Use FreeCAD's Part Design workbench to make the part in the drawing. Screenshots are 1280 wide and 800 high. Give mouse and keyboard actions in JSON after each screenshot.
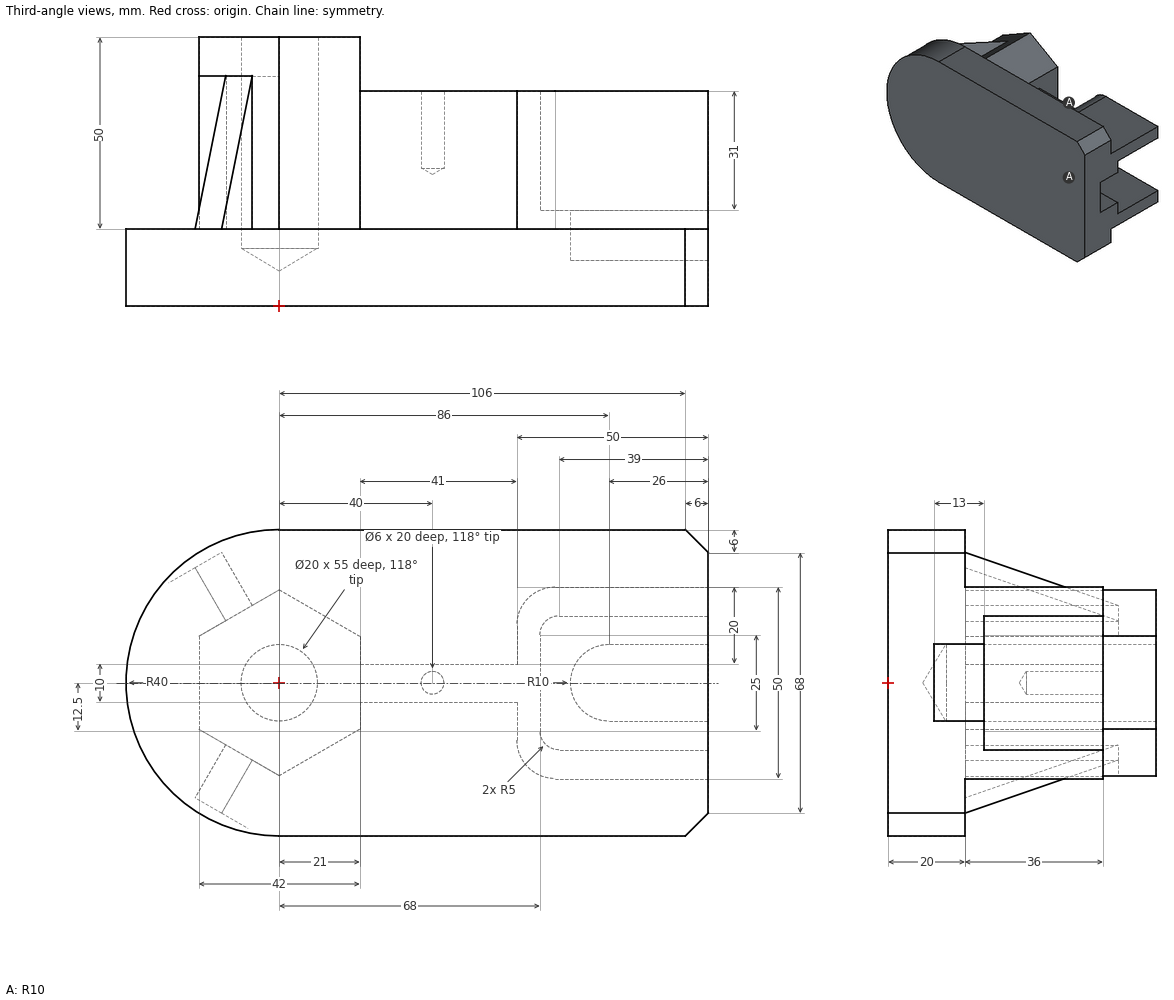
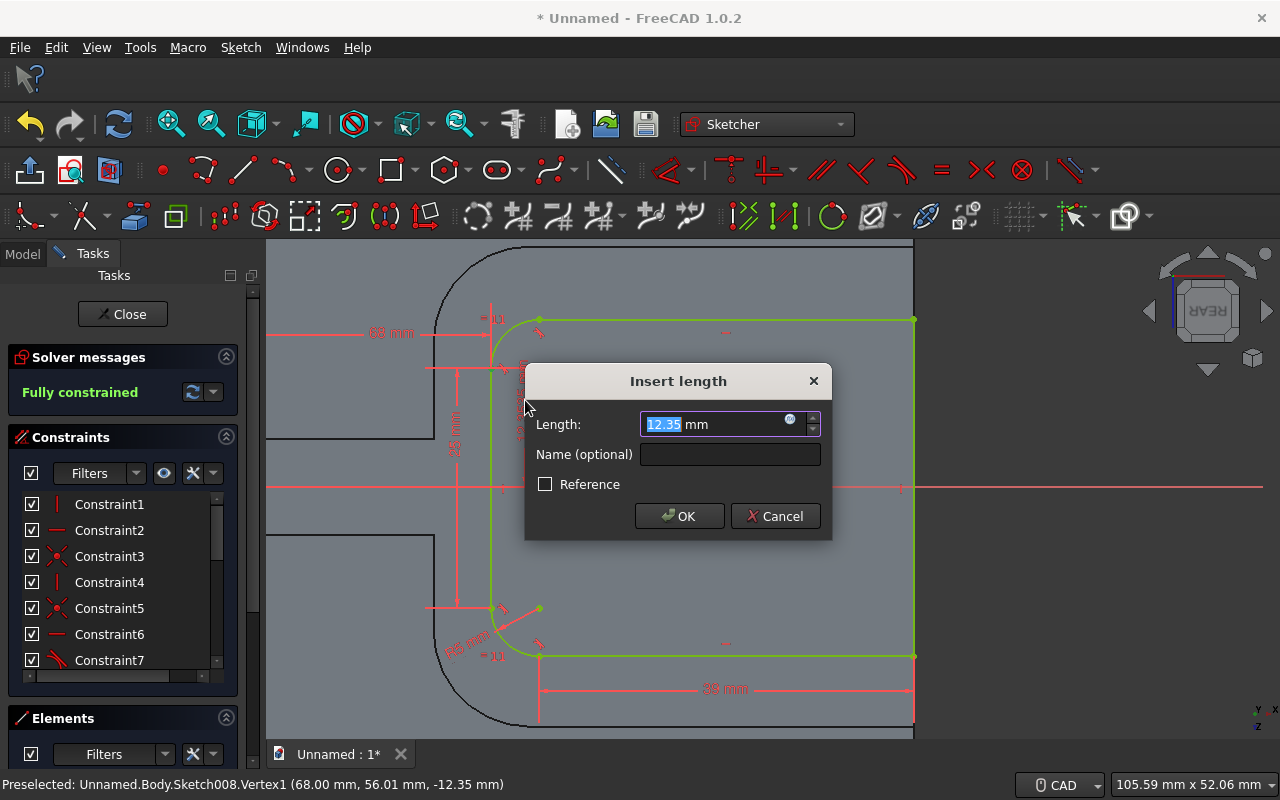
{"action": "type", "text": "12.5"}
{"action": "key", "text": "Return"}
{"action": "key", "text": "Escape"}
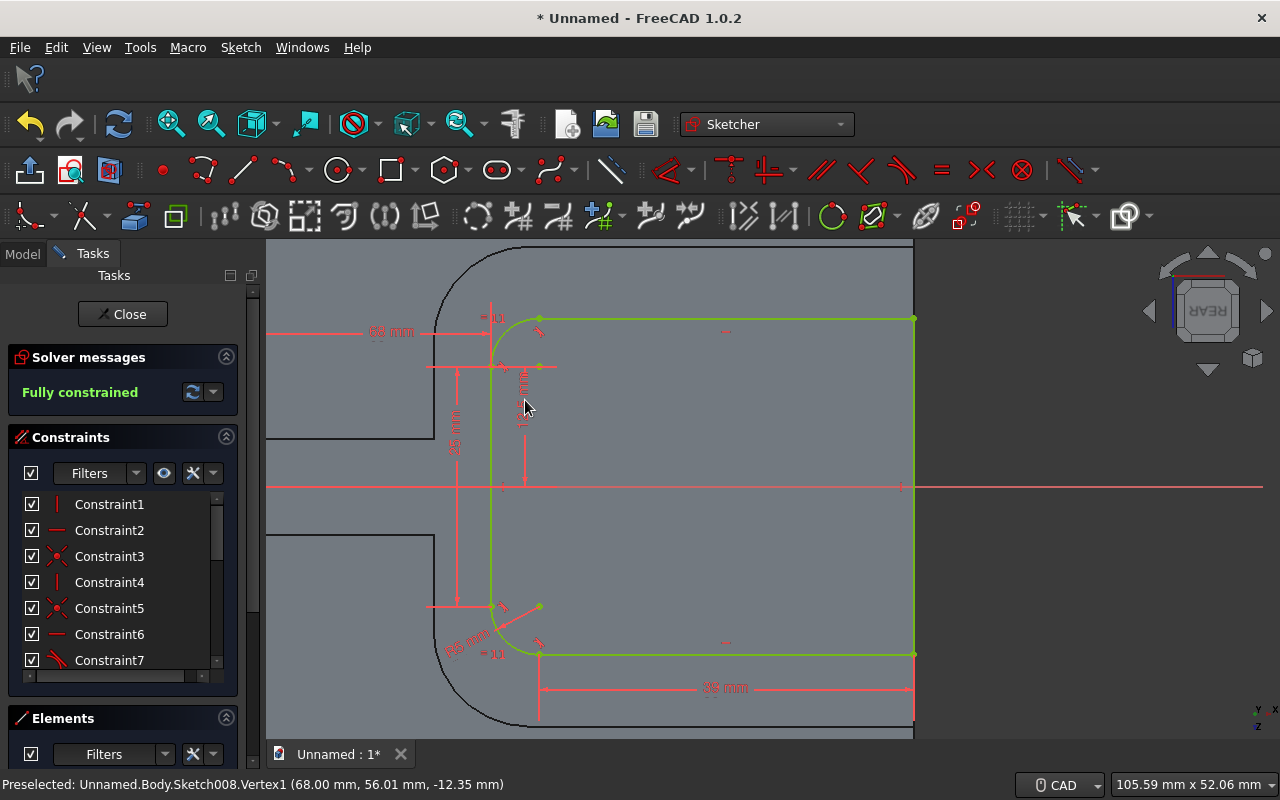
{"action": "left_click", "coordinate": [123, 314]}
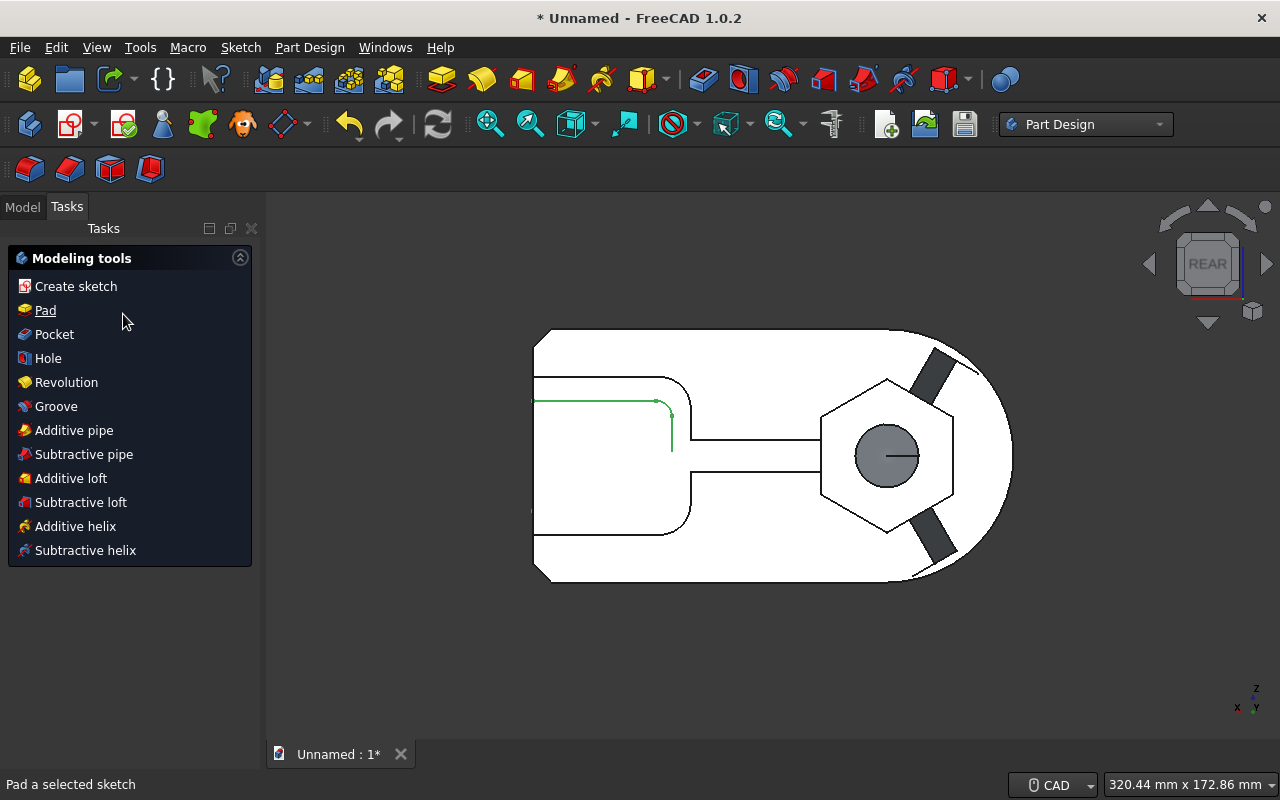
{"action": "left_click", "coordinate": [704, 80]}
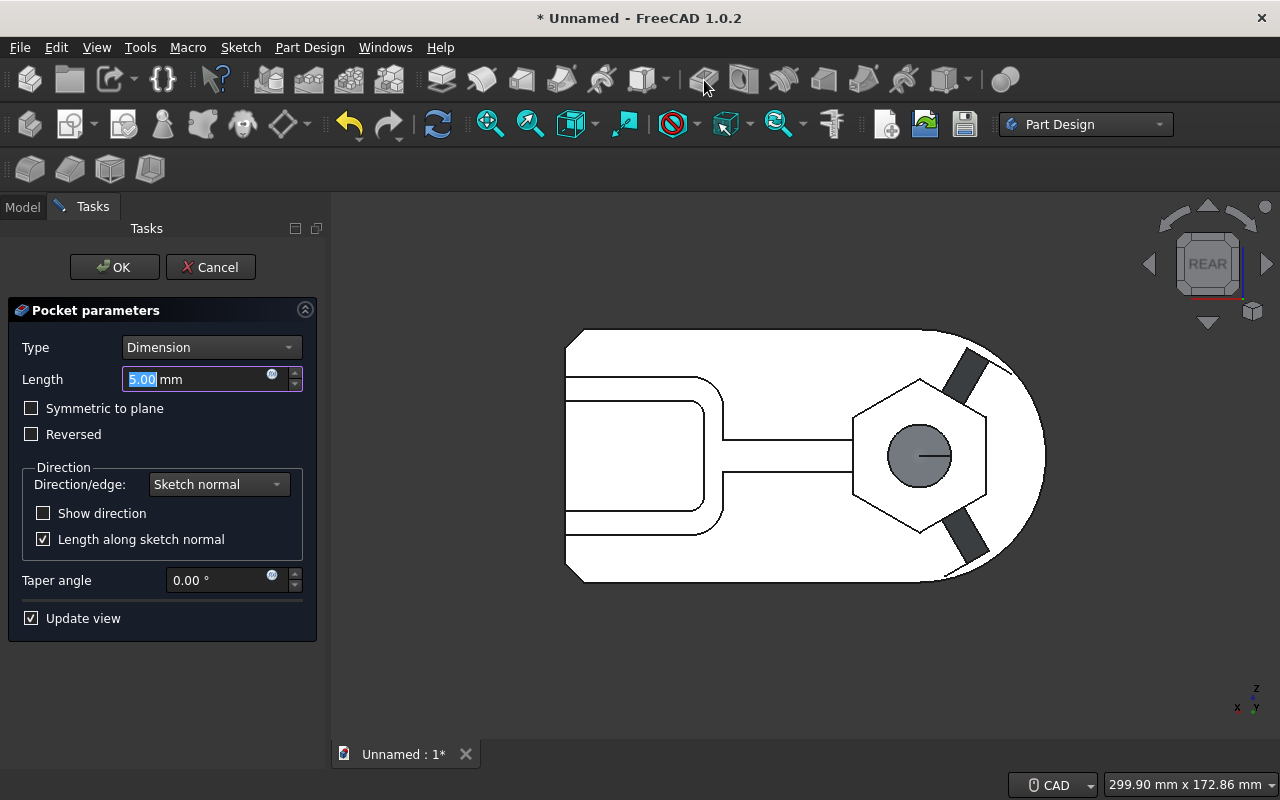
{"action": "type", "text": "31"}
{"action": "key", "text": "Tab"}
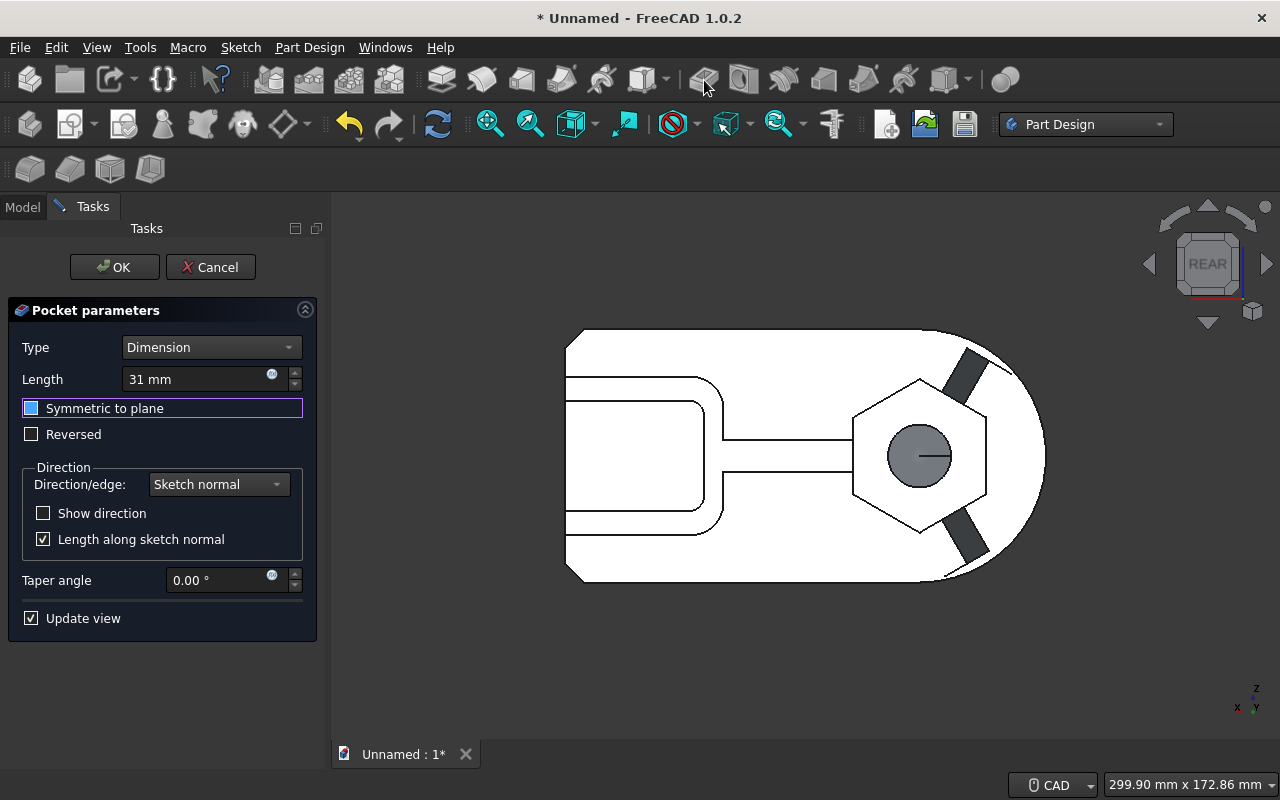
{"action": "left_click", "coordinate": [115, 267]}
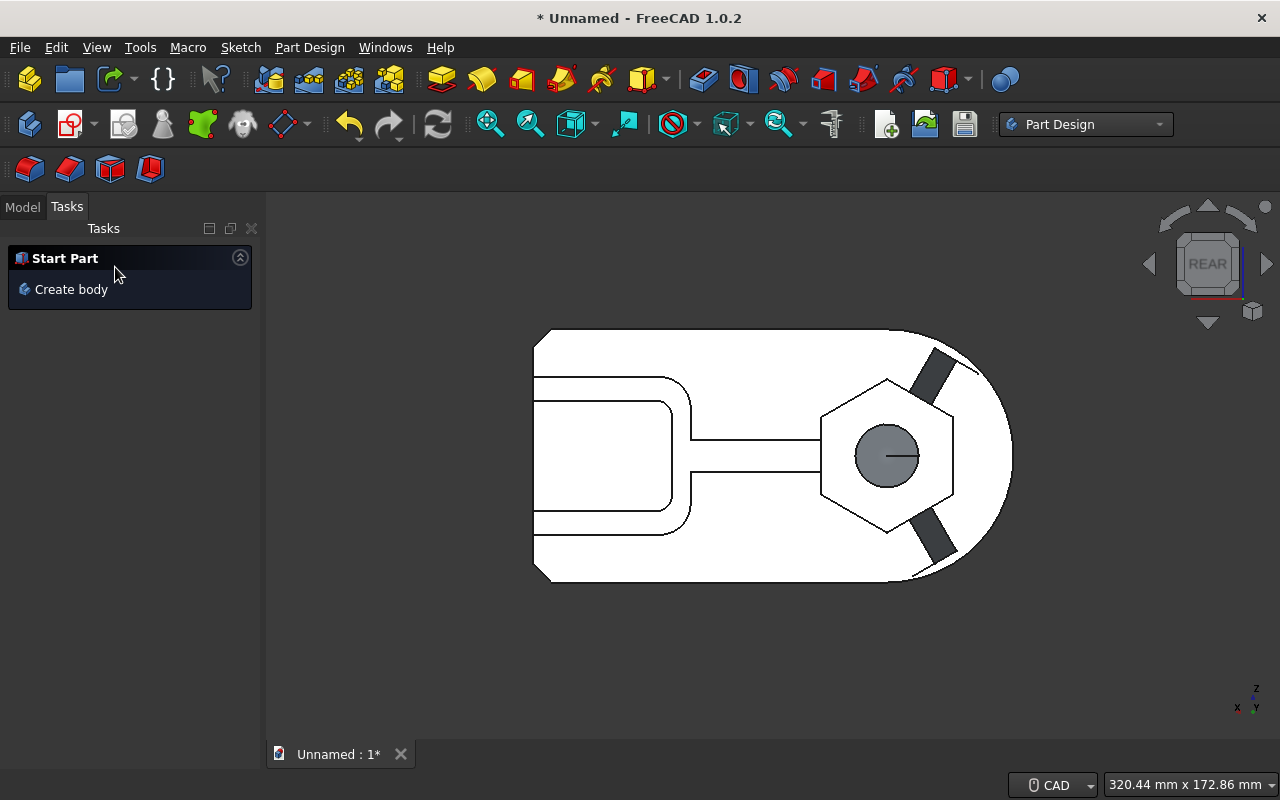
{"action": "left_click", "coordinate": [602, 455]}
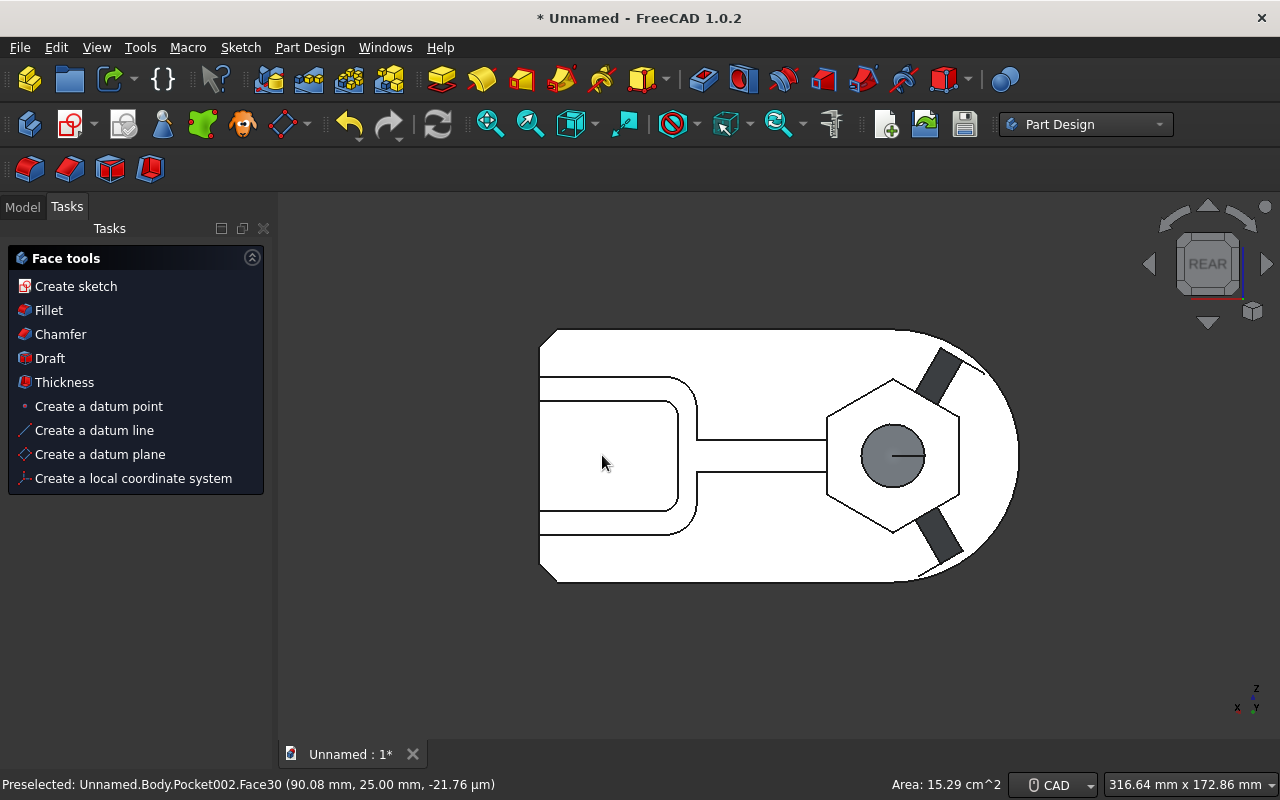
{"action": "left_click", "coordinate": [70, 124]}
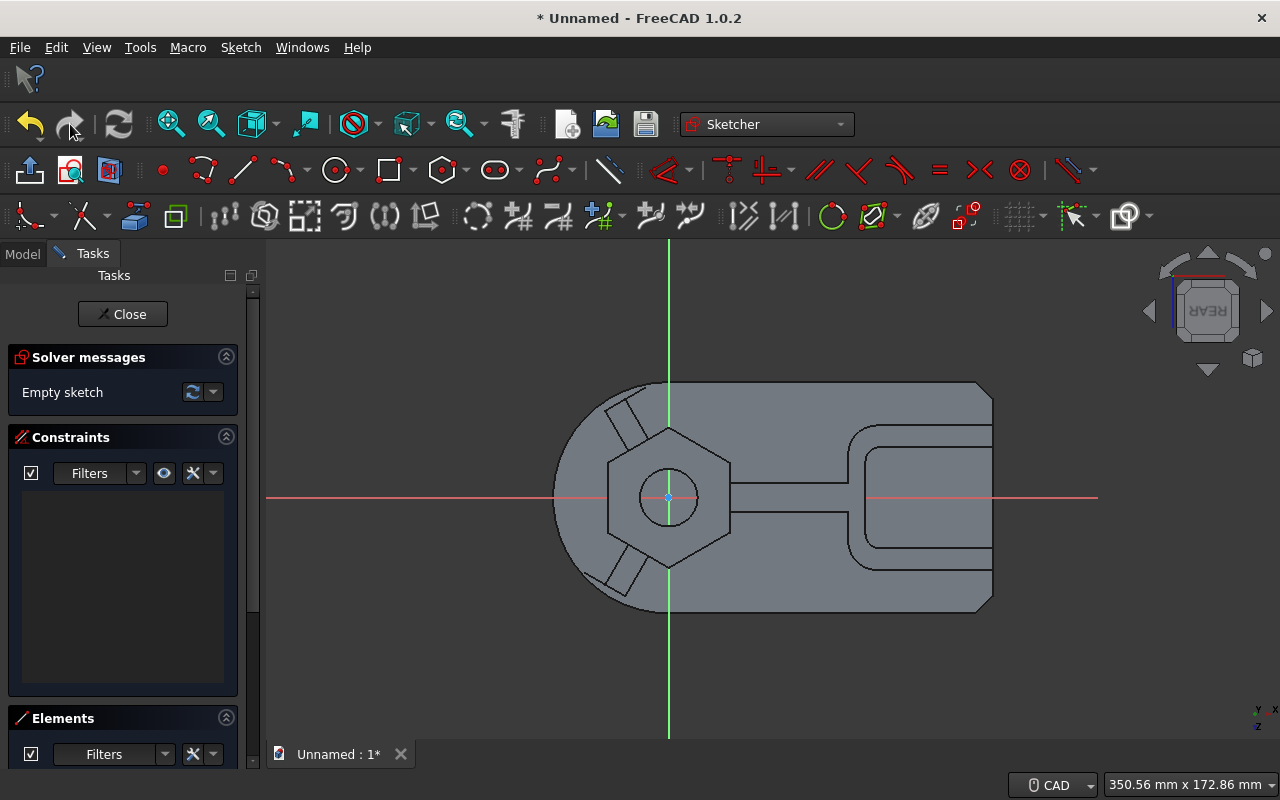
{"action": "left_click", "coordinate": [110, 170]}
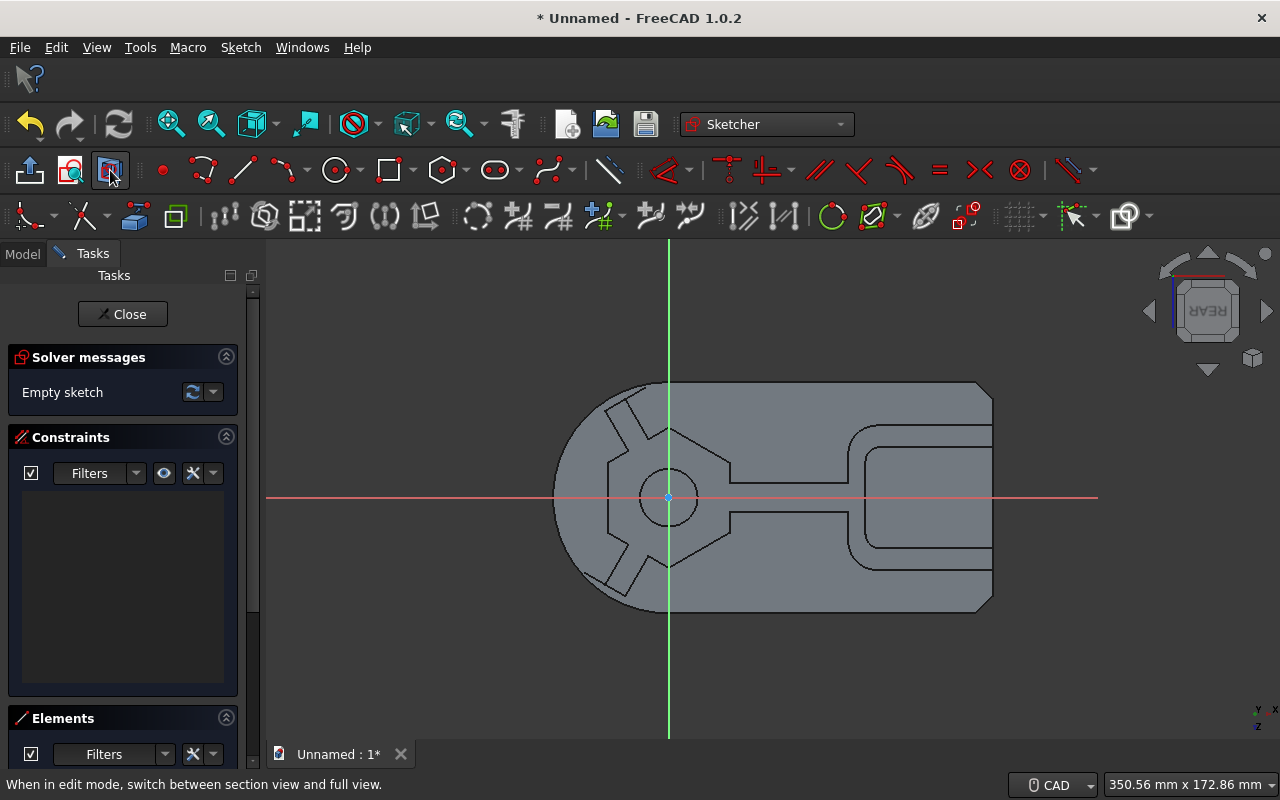
{"action": "scroll", "coordinate": [1000, 500], "scroll_direction": "up", "scroll_amount": 8}